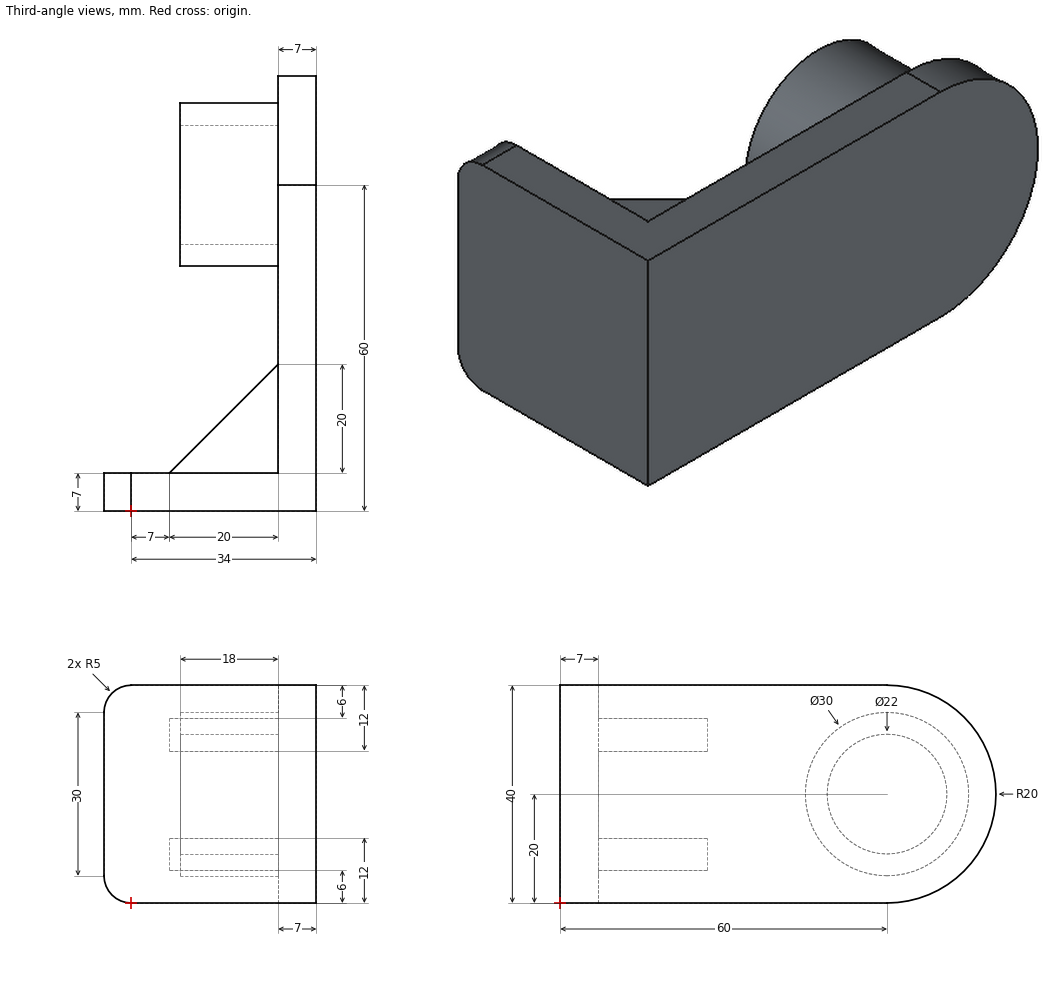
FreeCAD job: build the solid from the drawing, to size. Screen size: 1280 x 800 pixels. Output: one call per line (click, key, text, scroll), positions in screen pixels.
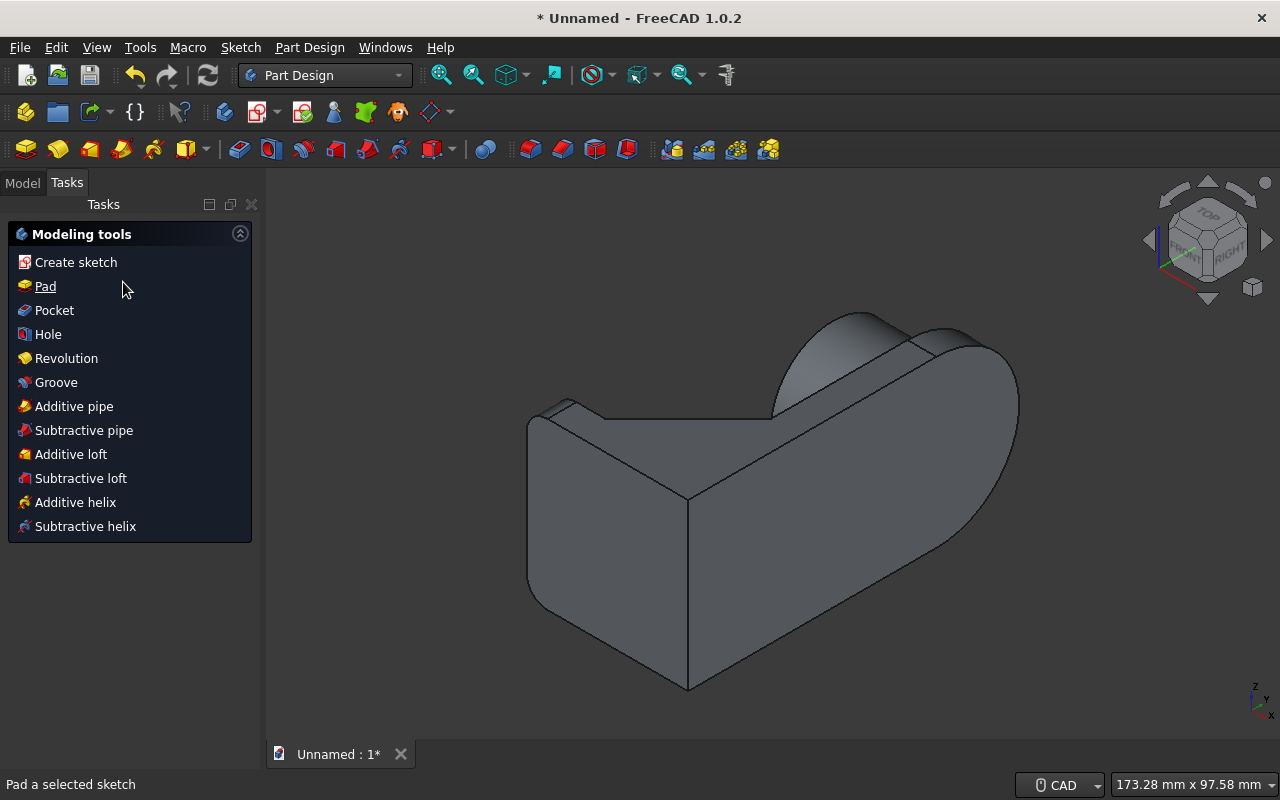
click(240, 150)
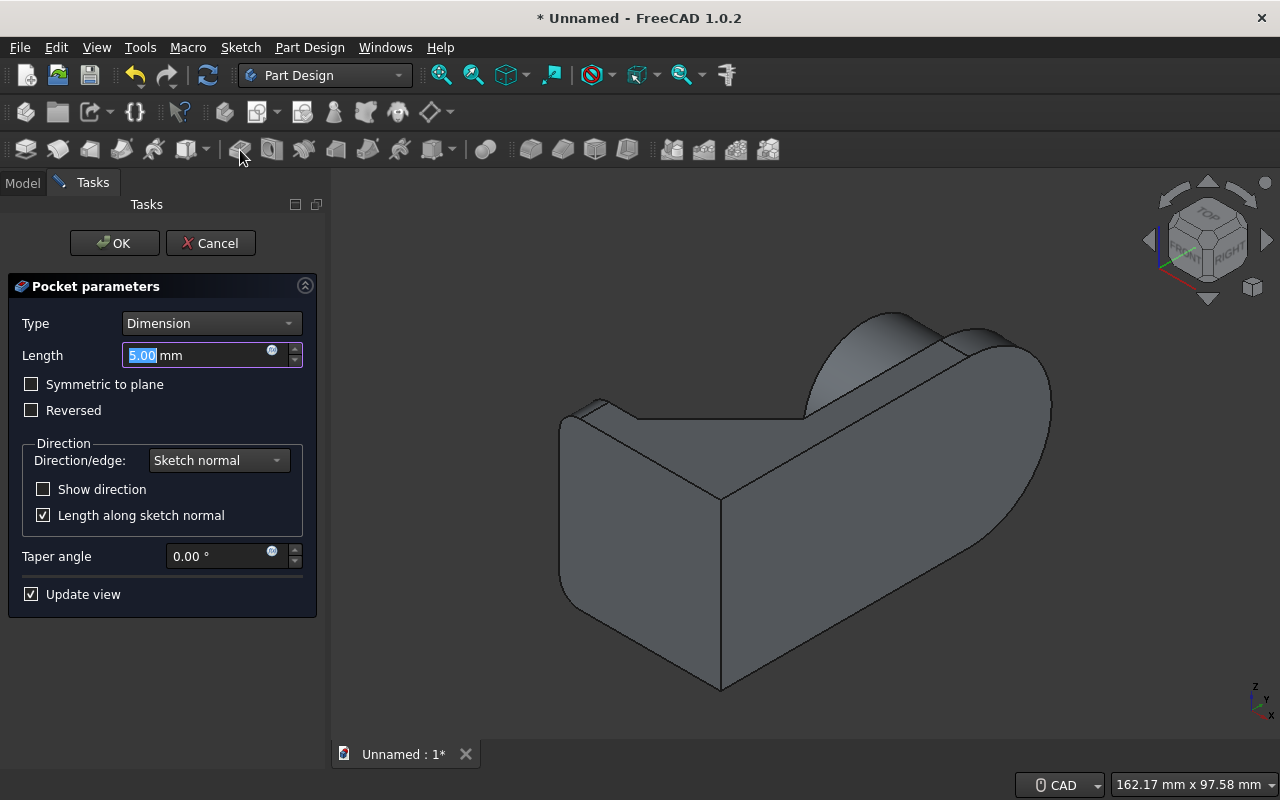
text(6)
key(Tab)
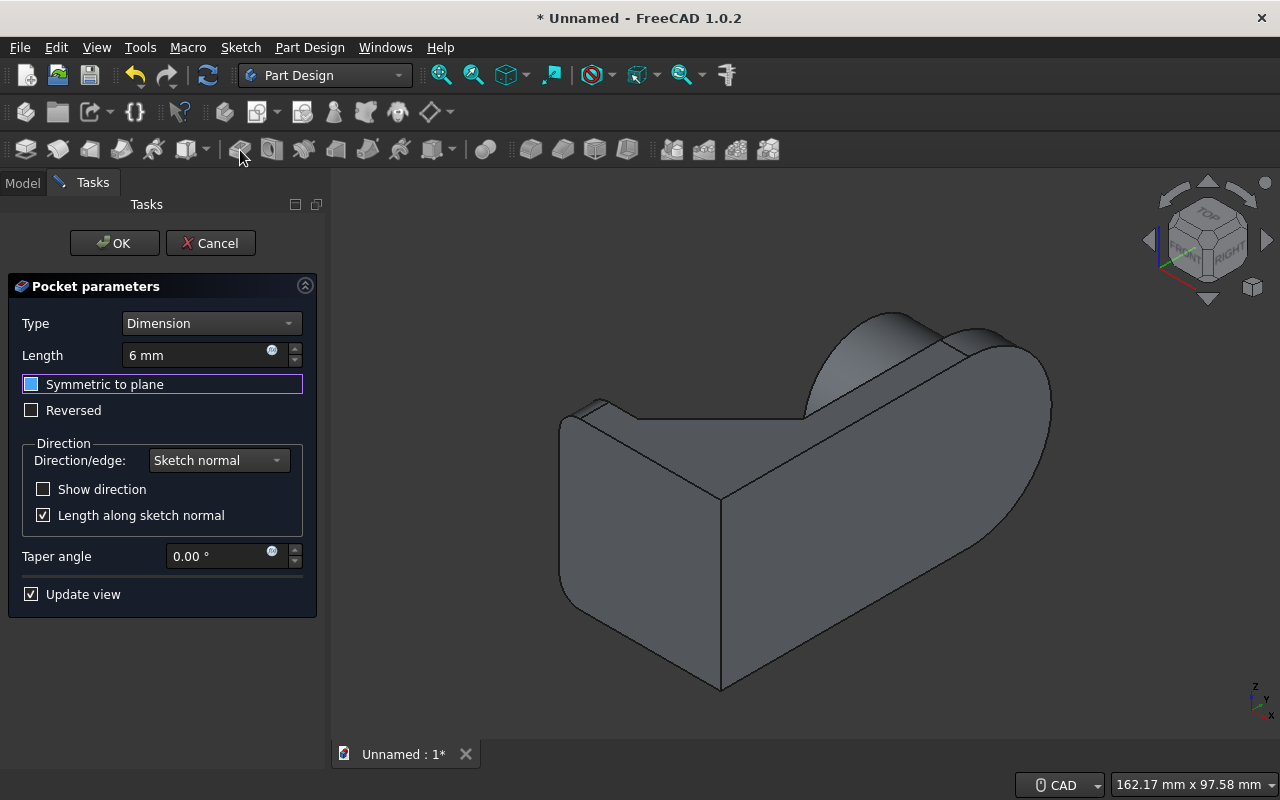
click(30, 410)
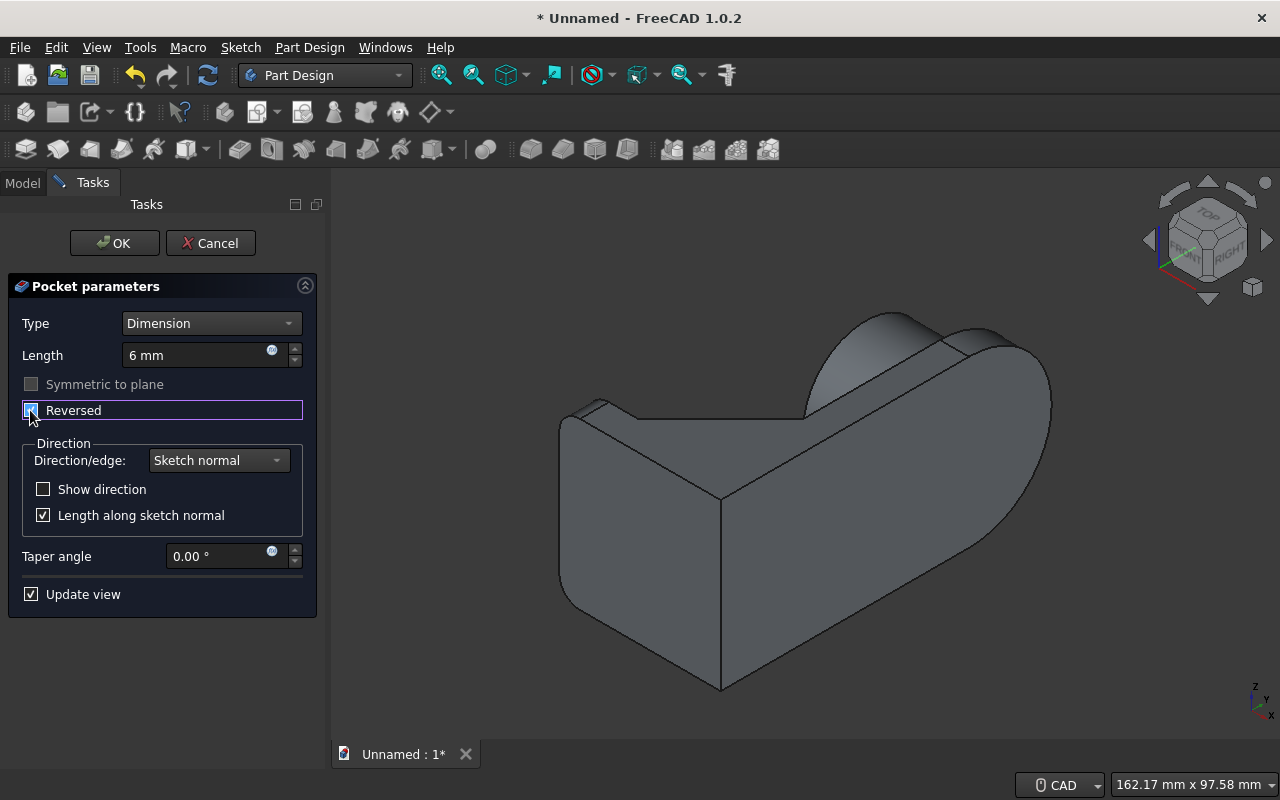
click(115, 243)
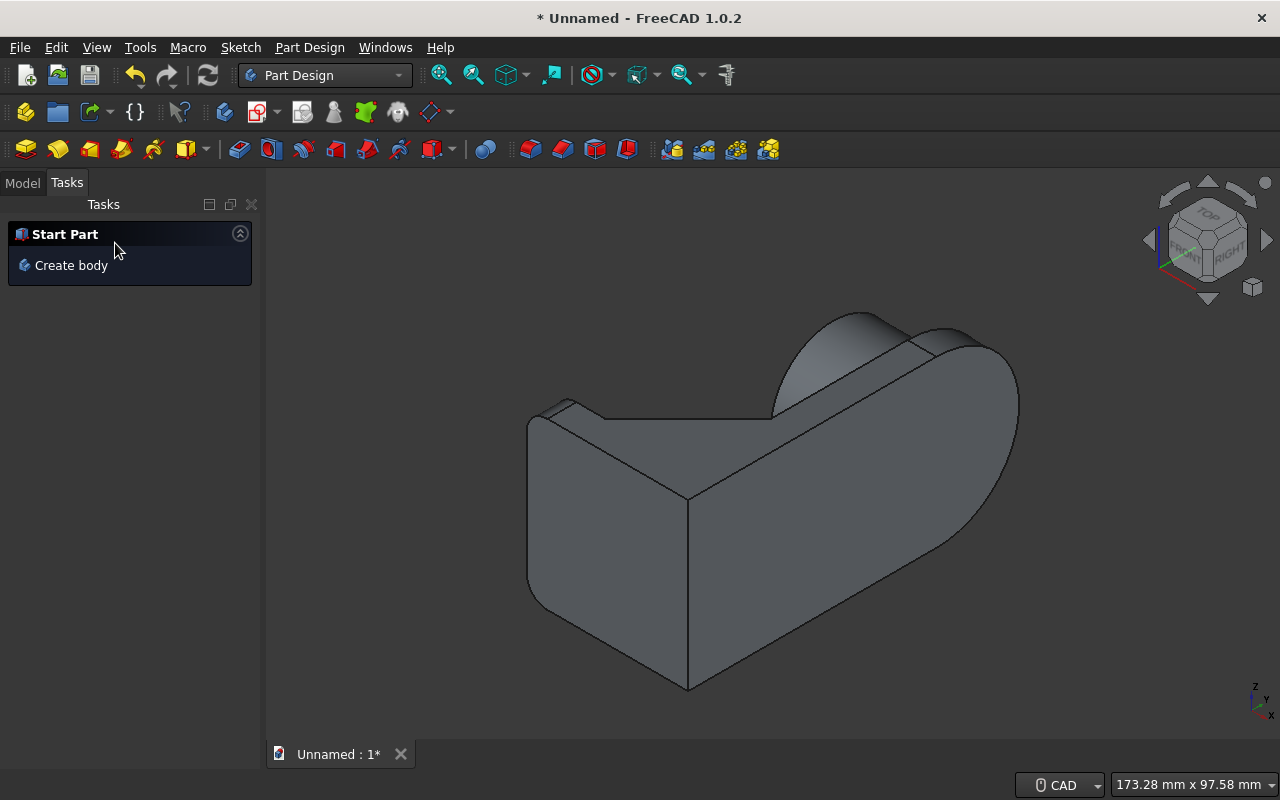
click(711, 451)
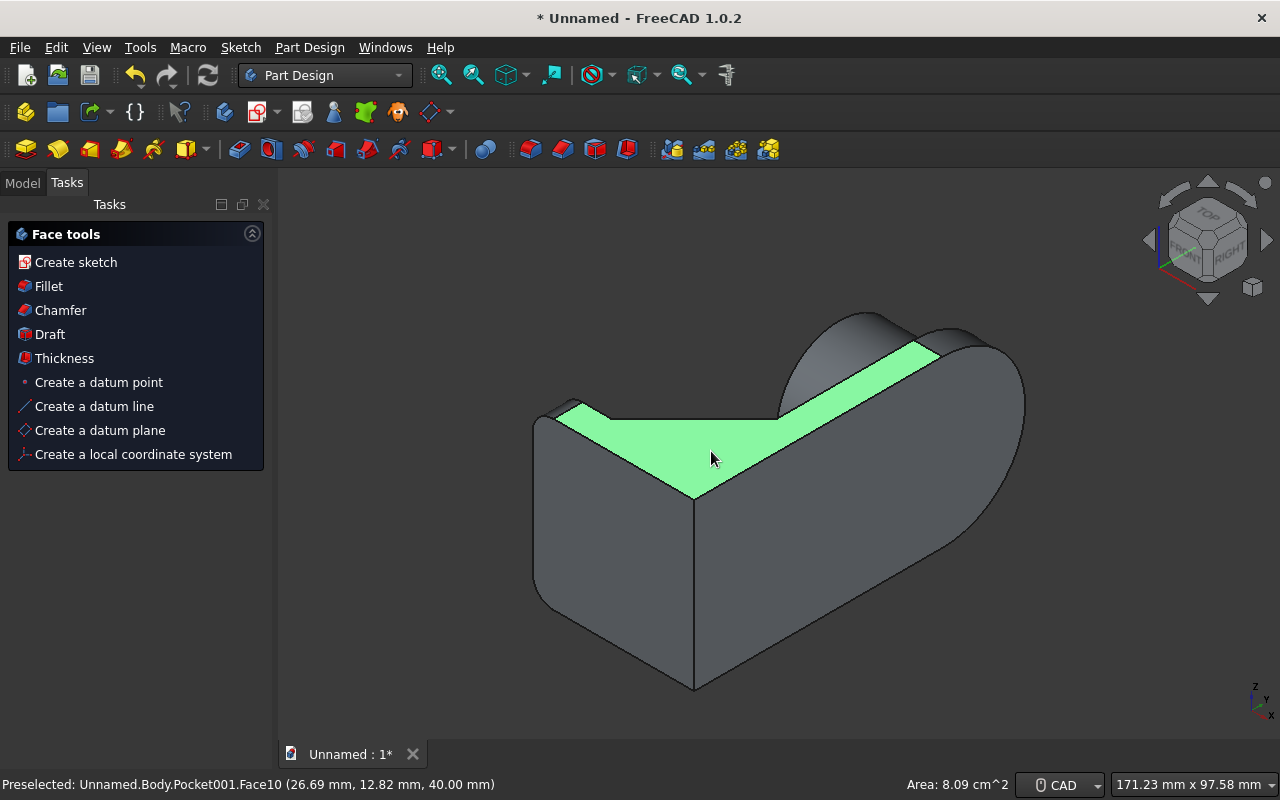
click(258, 112)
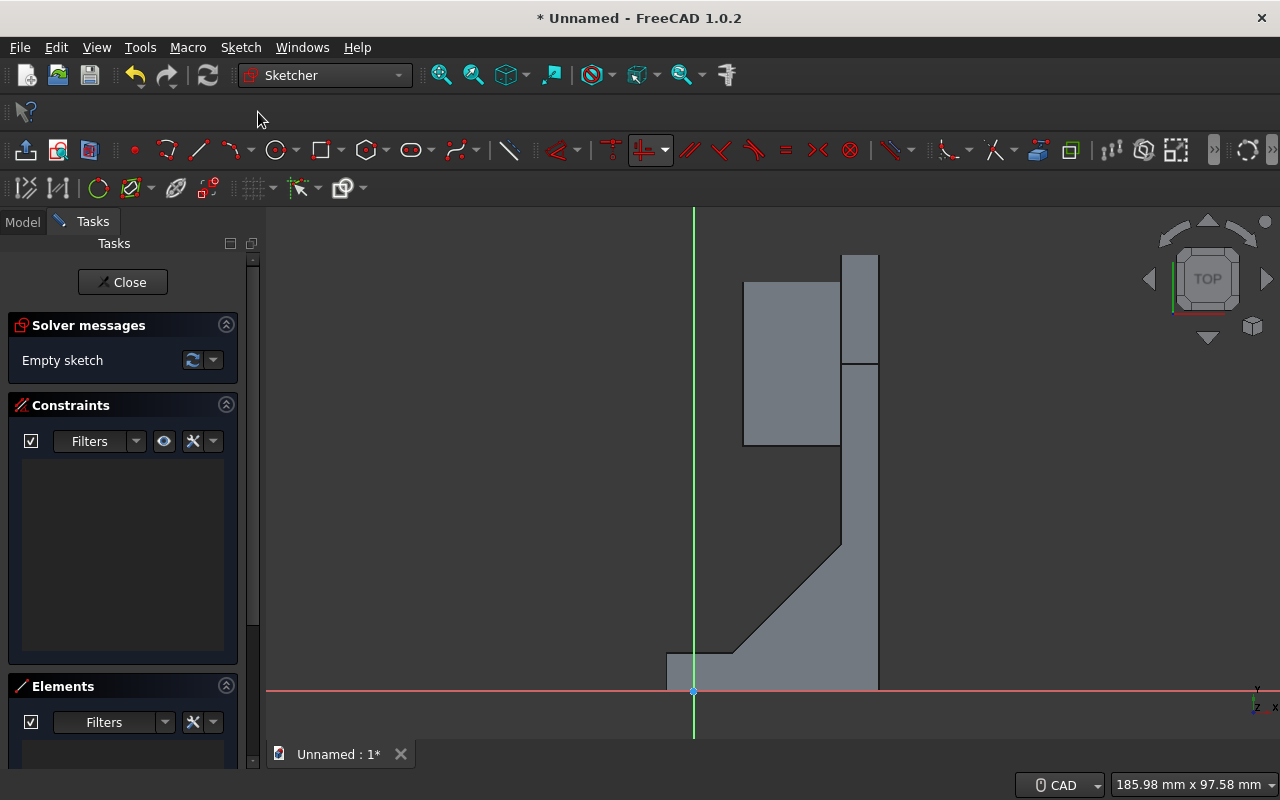
scroll(819, 711, up, 4)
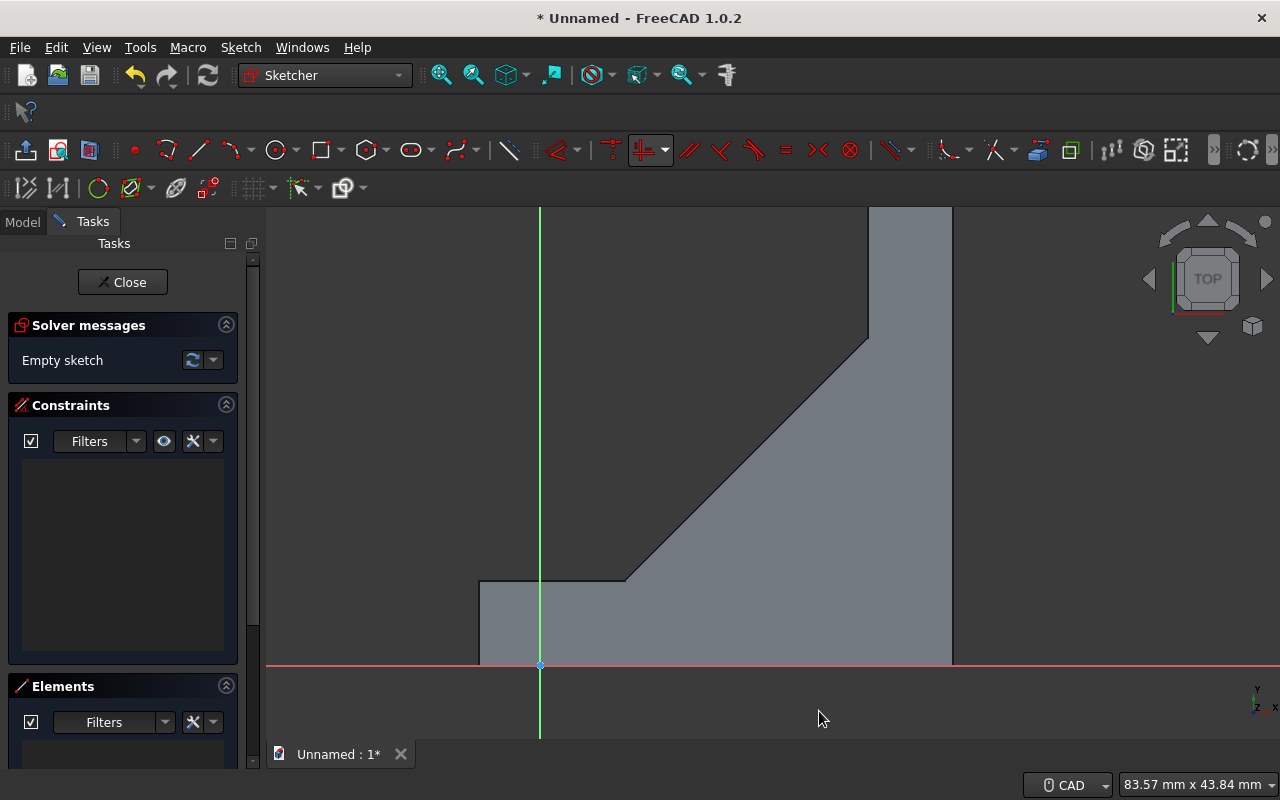
click(168, 150)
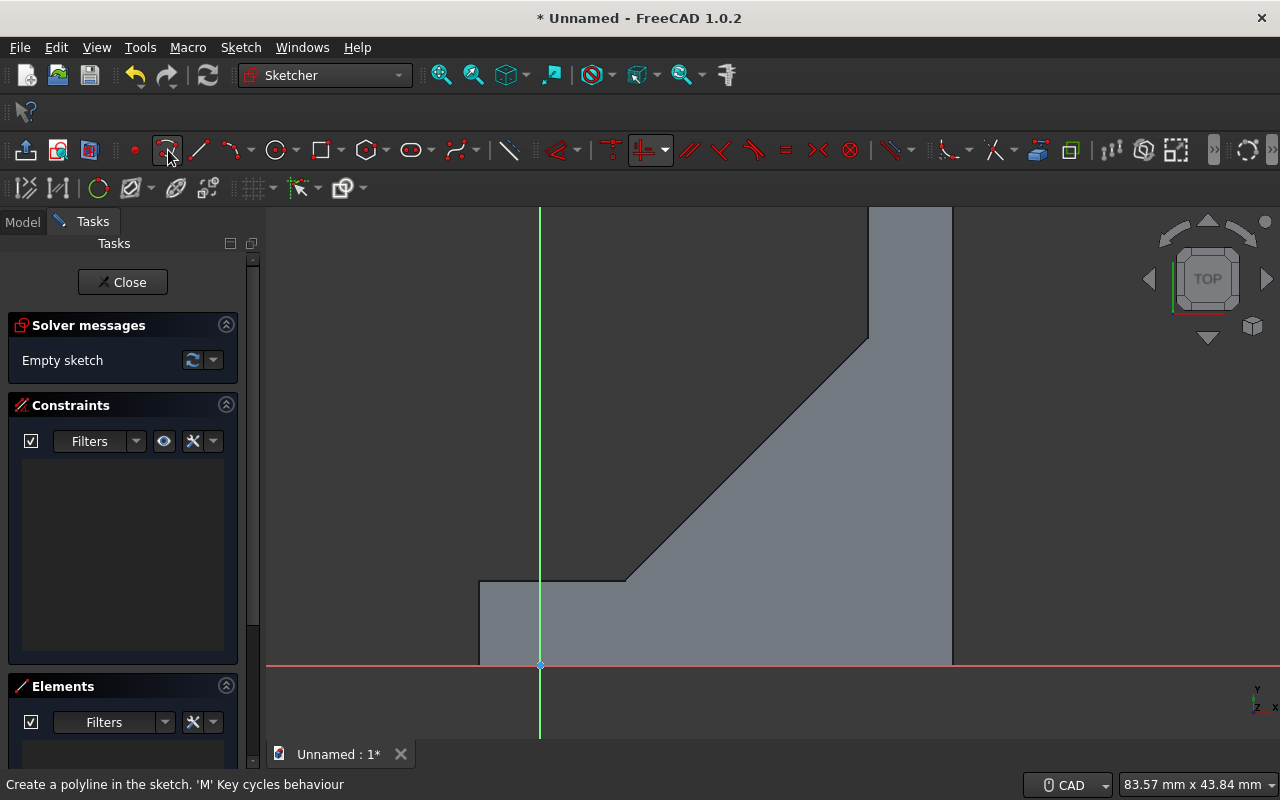
click(625, 581)
click(868, 581)
click(868, 338)
click(625, 582)
key(Escape)
key(Escape)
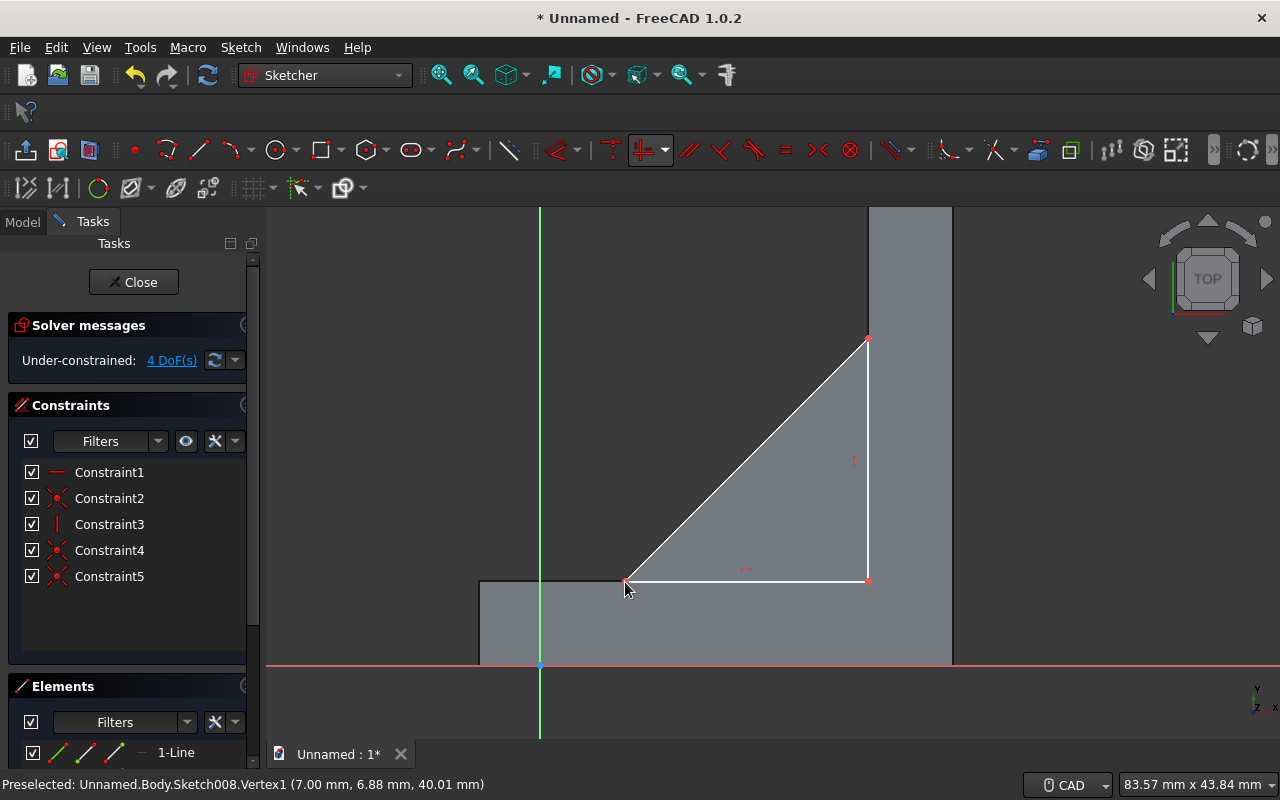
click(556, 150)